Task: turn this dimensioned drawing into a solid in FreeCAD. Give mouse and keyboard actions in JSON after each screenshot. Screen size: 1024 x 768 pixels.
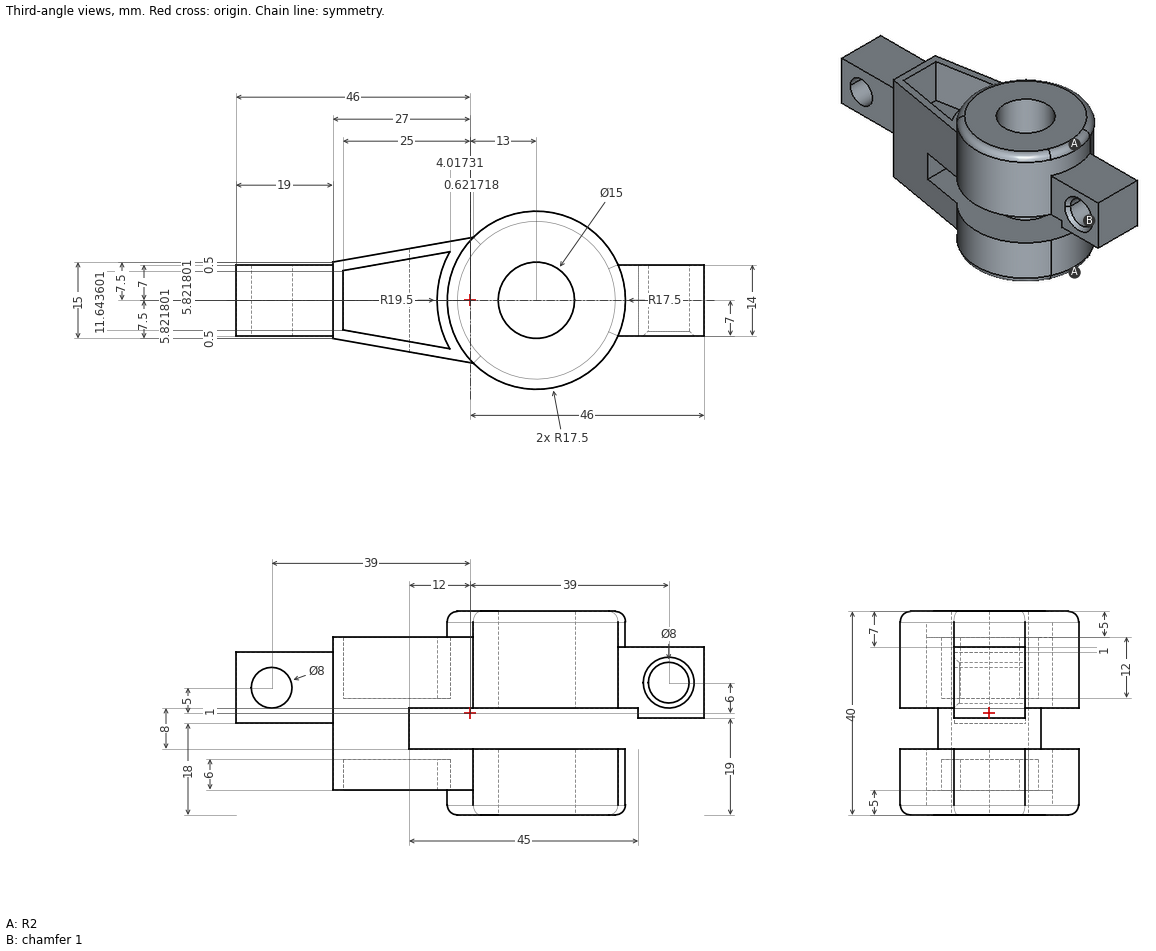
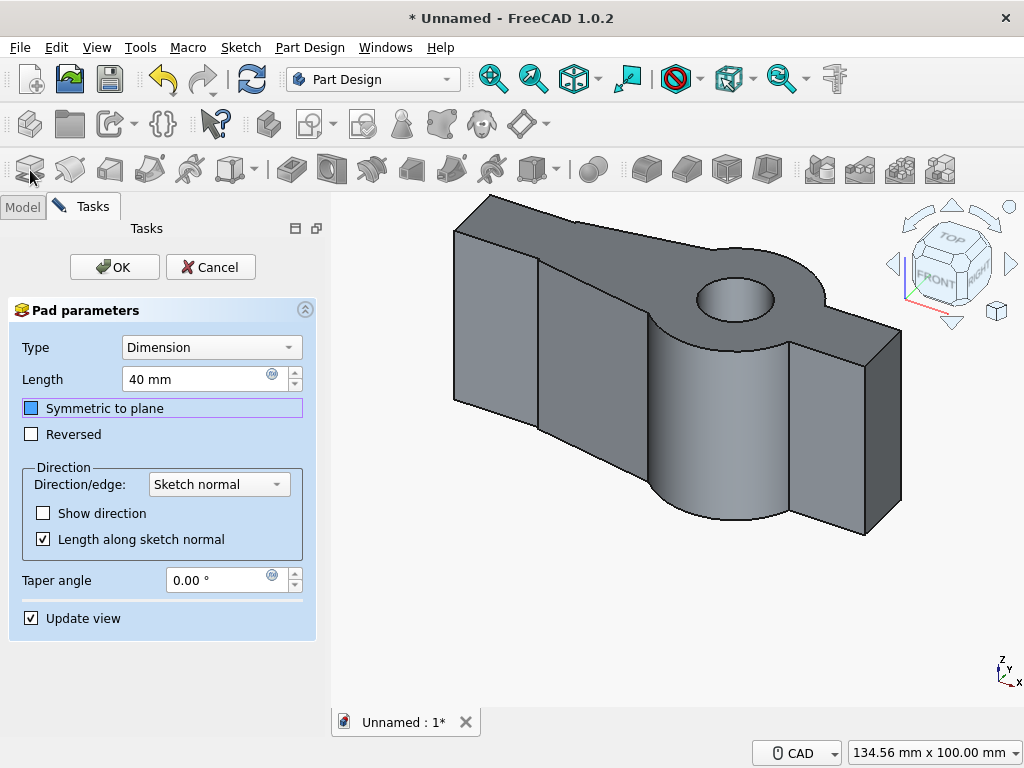
{"action": "left_click", "coordinate": [30, 408]}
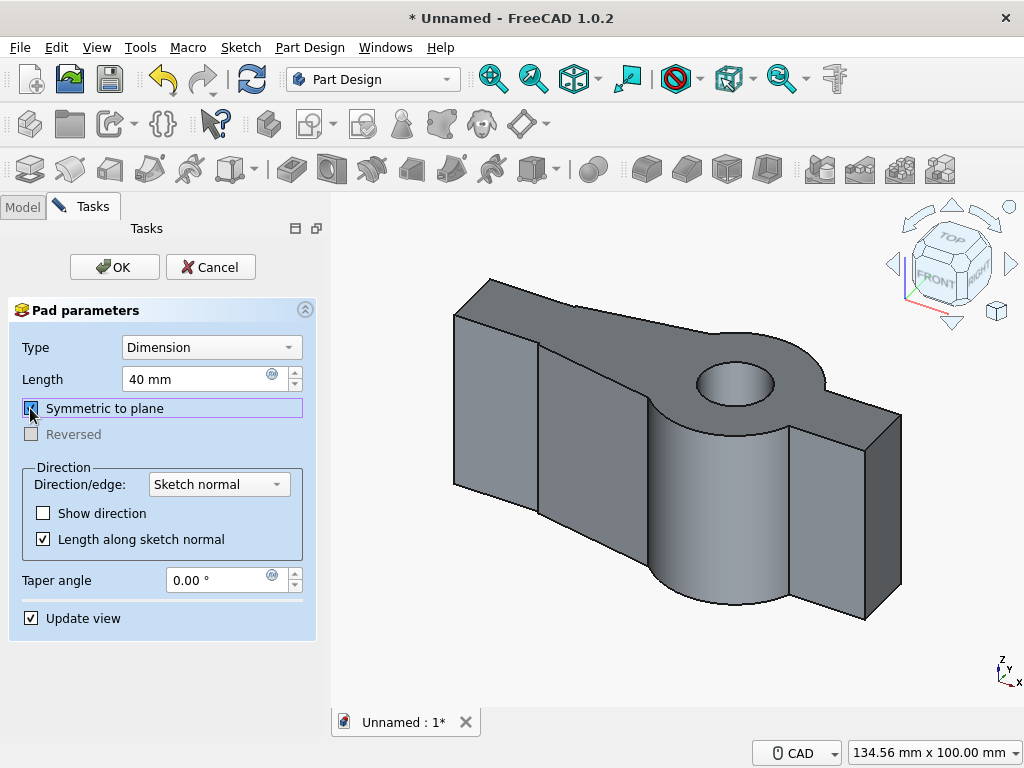
{"action": "left_click", "coordinate": [115, 267]}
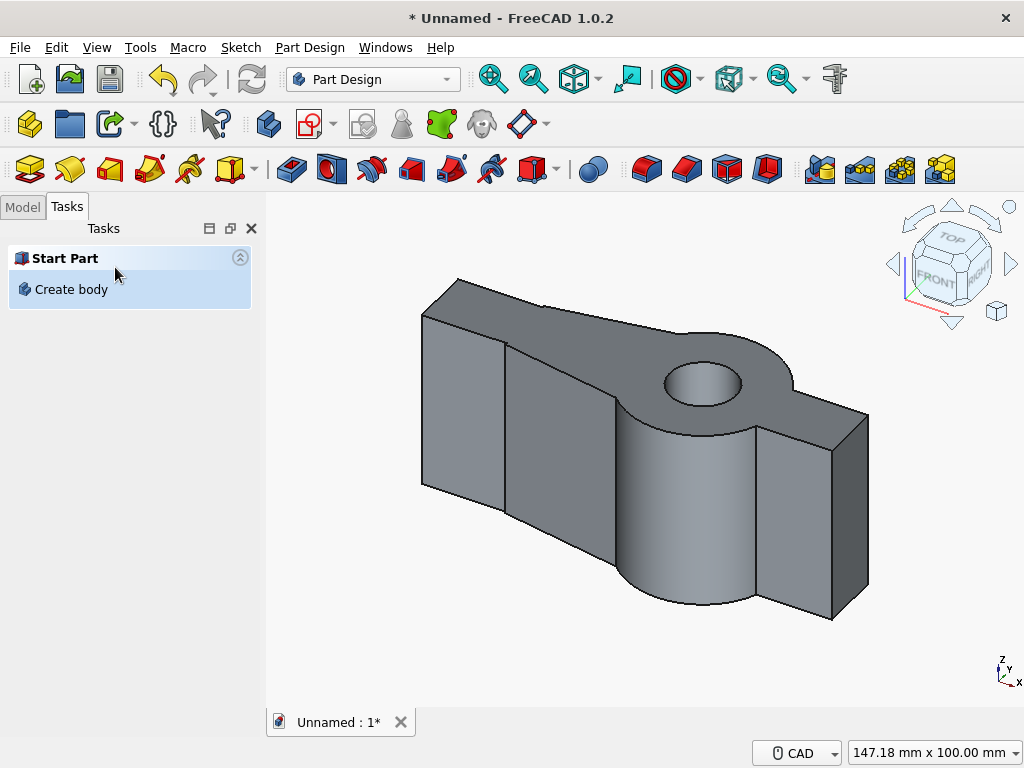
{"action": "left_click", "coordinate": [310, 124]}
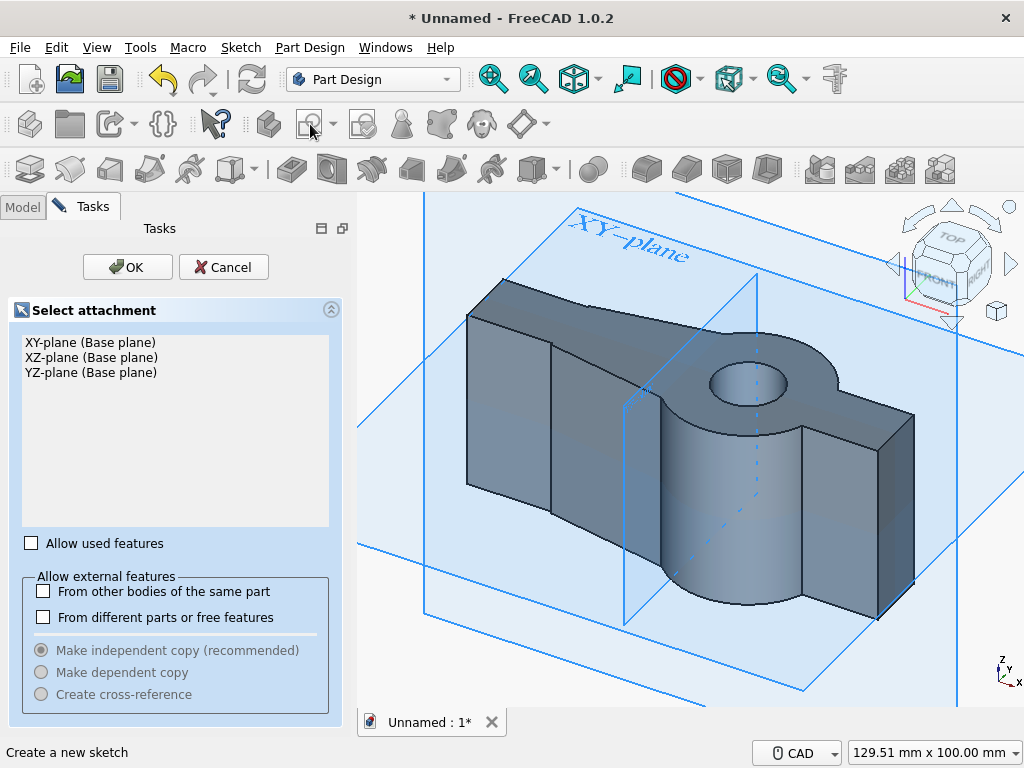
{"action": "left_click", "coordinate": [82, 358]}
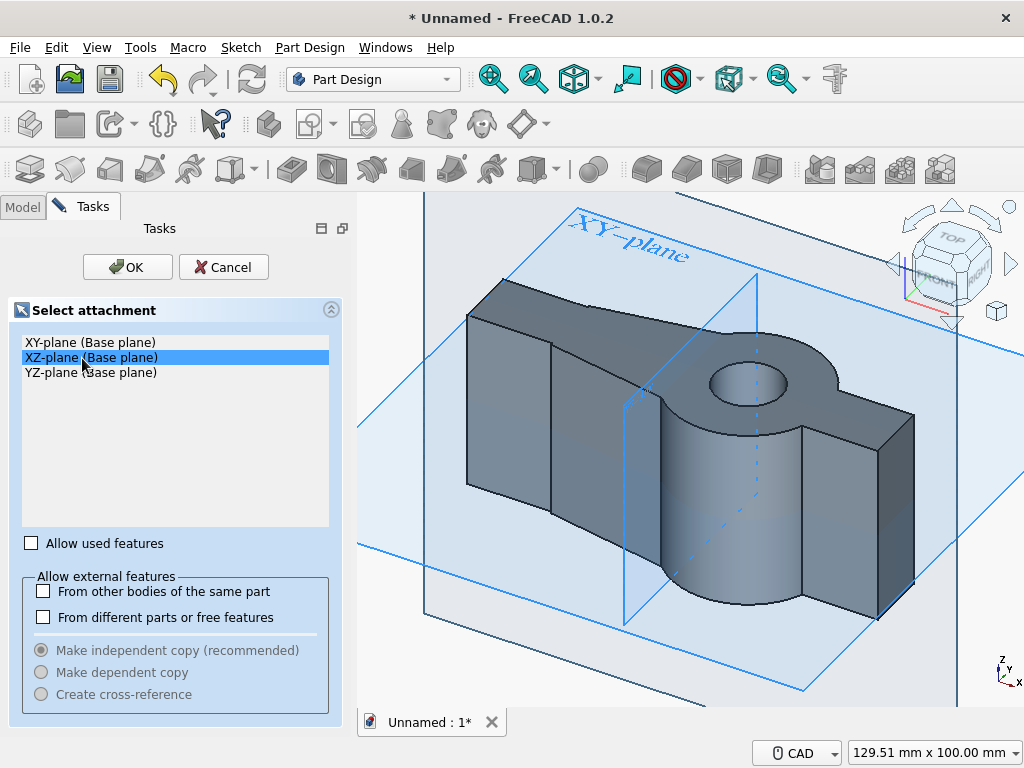
{"action": "left_click", "coordinate": [128, 267]}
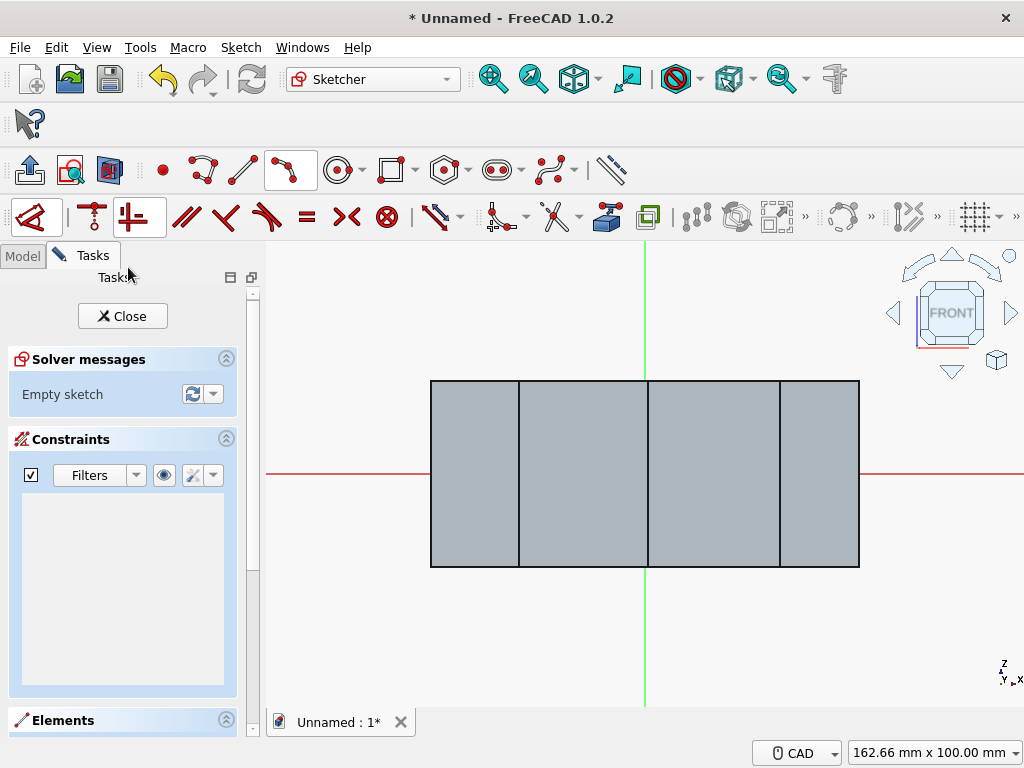
{"action": "left_click", "coordinate": [110, 170]}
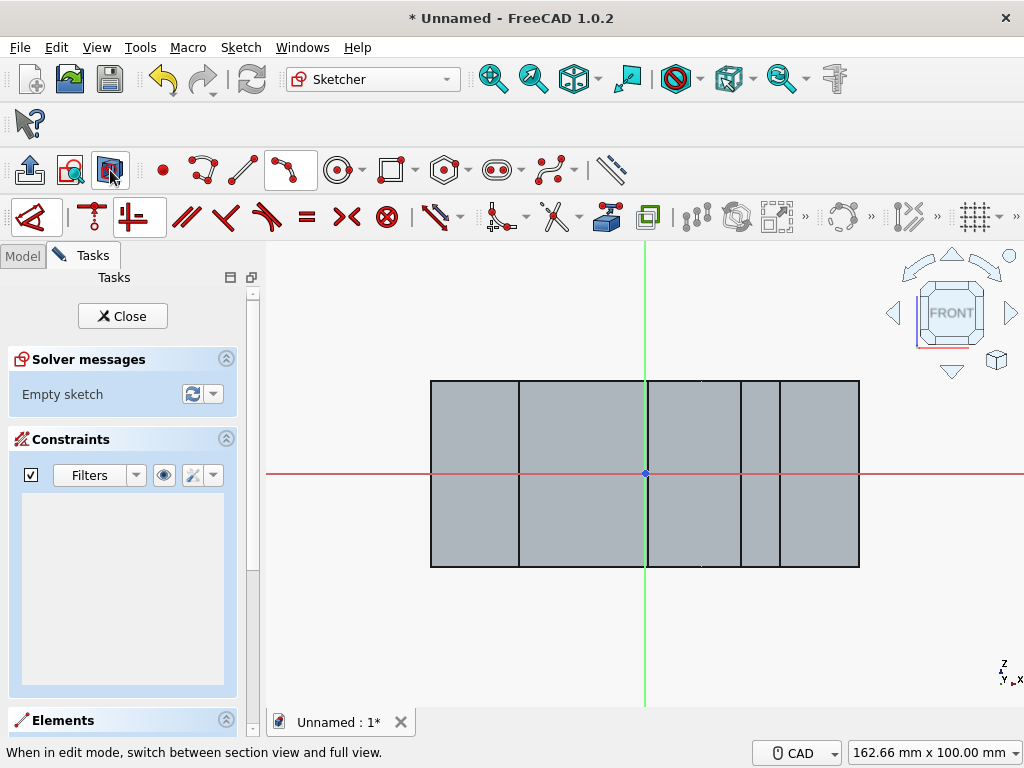
{"action": "scroll", "coordinate": [837, 505], "scroll_direction": "up", "scroll_amount": 3}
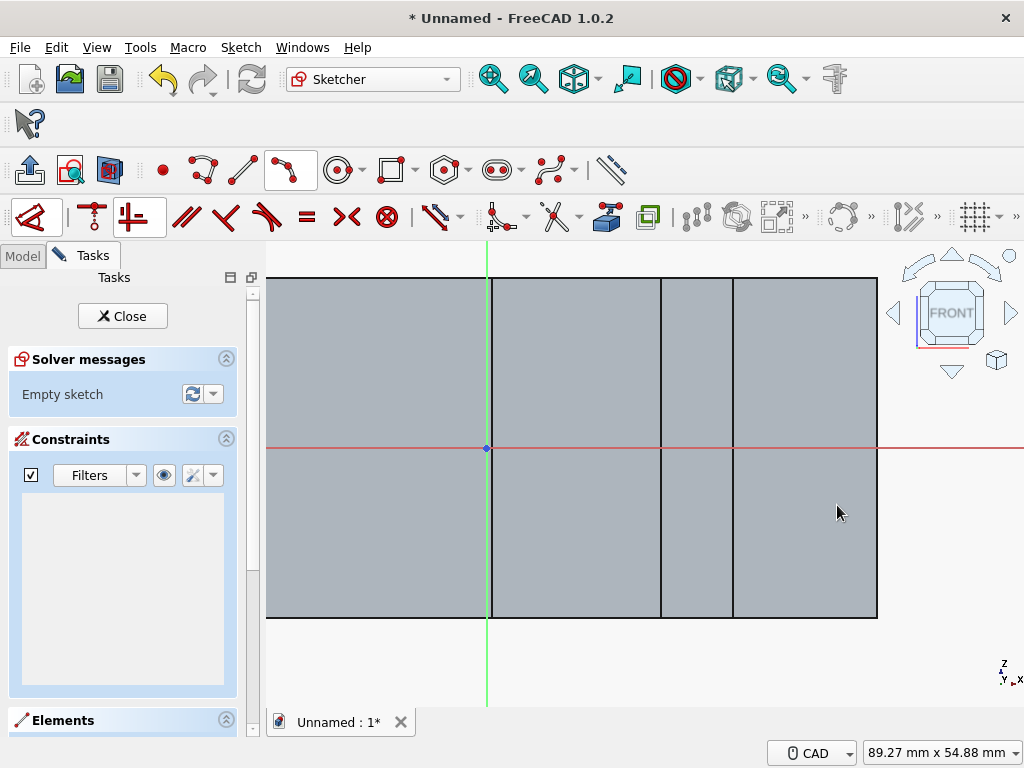
{"action": "left_click", "coordinate": [392, 170]}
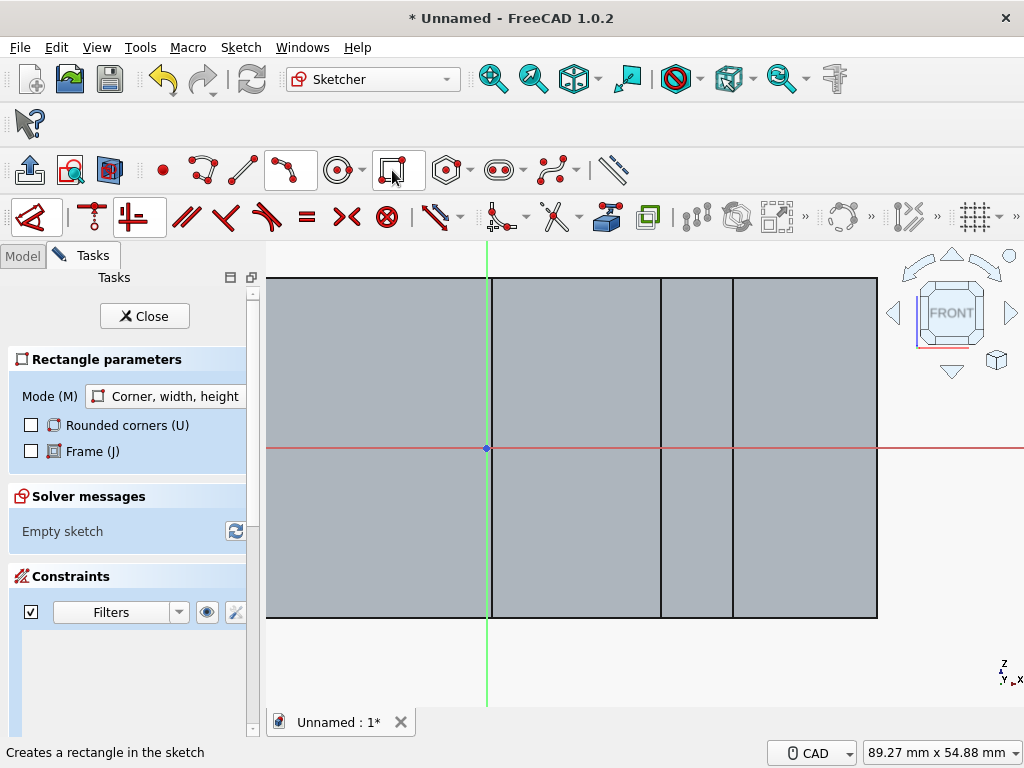
{"action": "scroll", "coordinate": [385, 440], "scroll_direction": "up", "scroll_amount": 4}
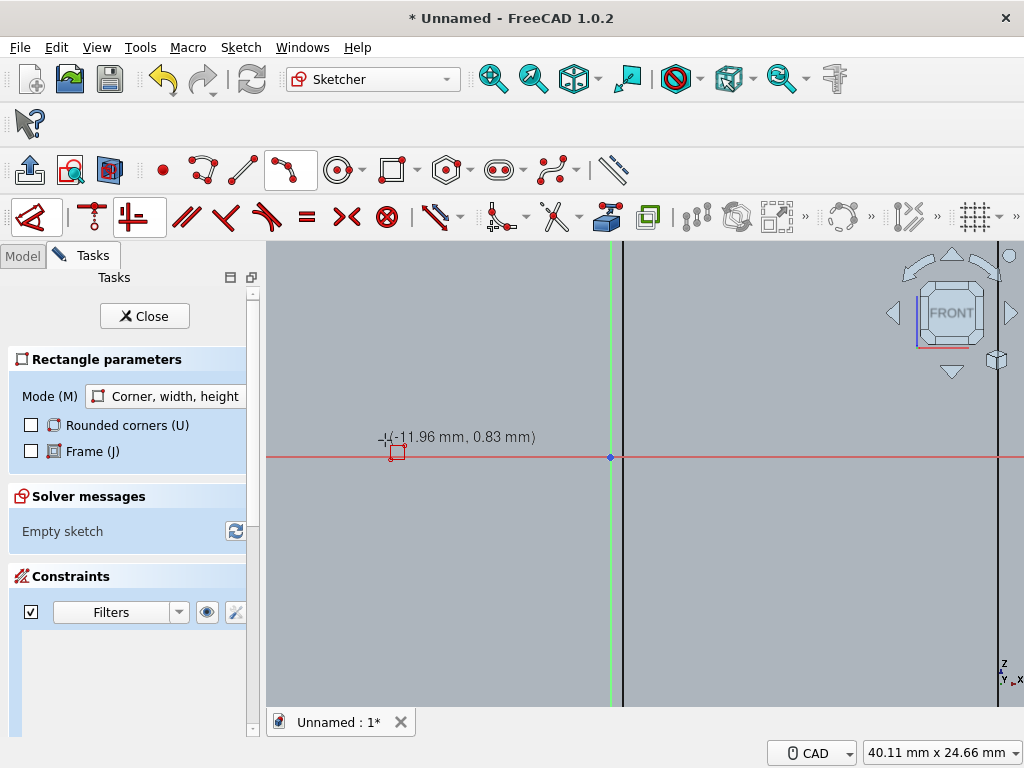
{"action": "left_click", "coordinate": [384, 438]}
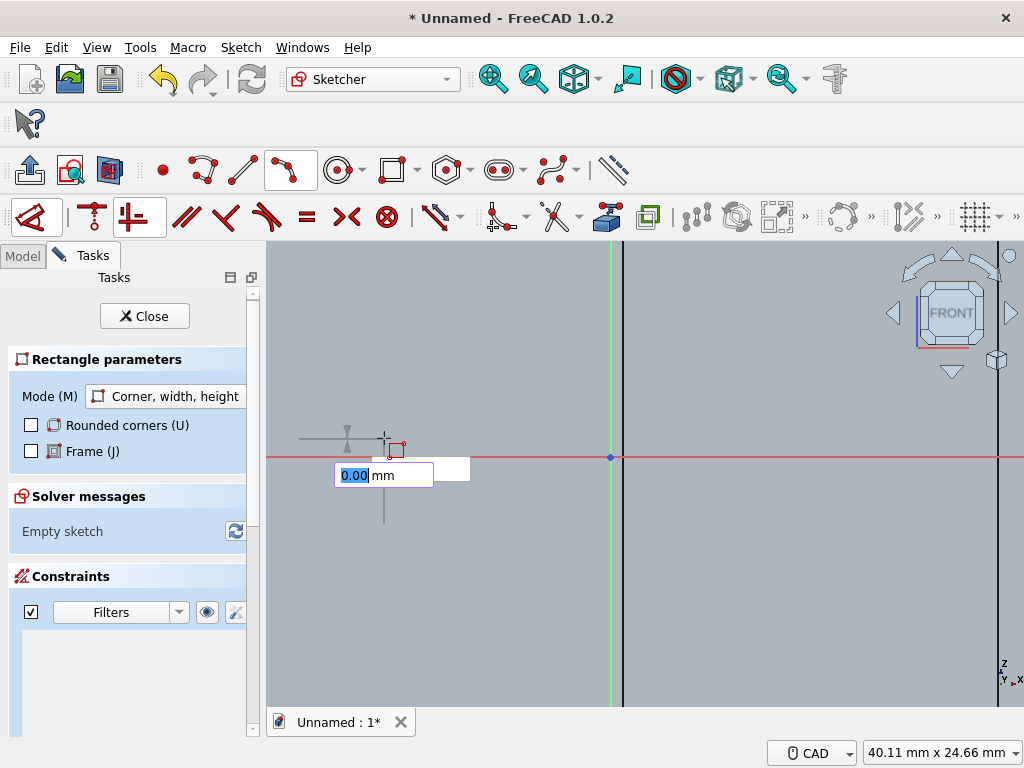
{"action": "scroll", "coordinate": [387, 441], "scroll_direction": "down", "scroll_amount": 4}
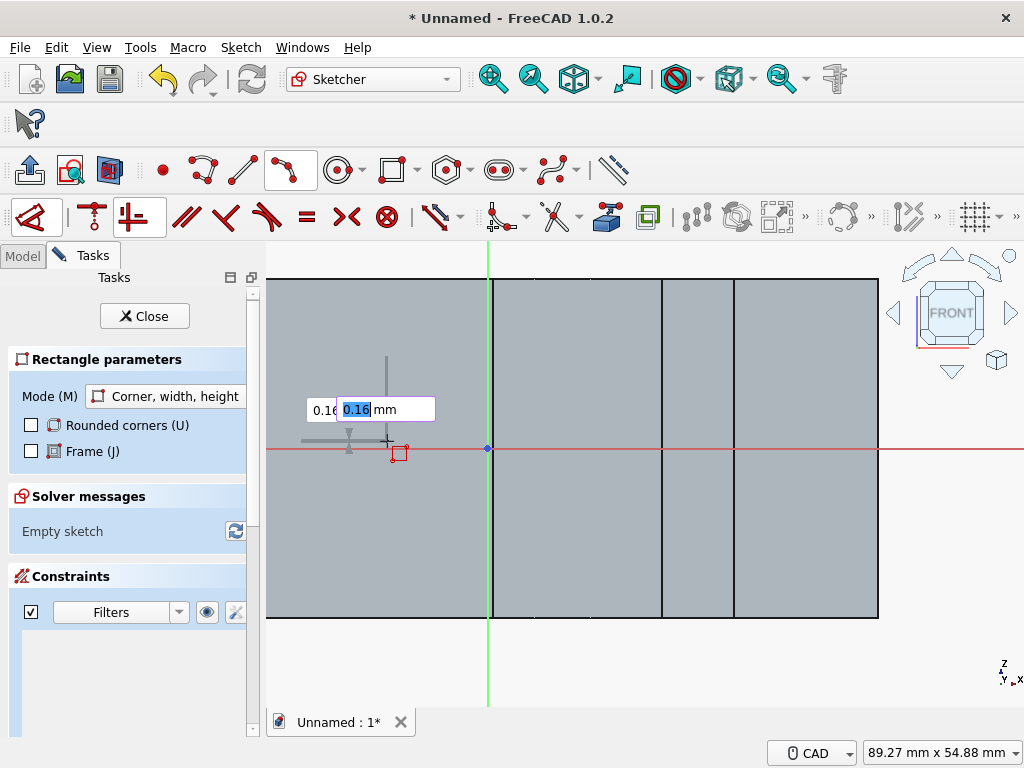
{"action": "left_click", "coordinate": [768, 508]}
{"action": "key", "text": "Escape"}